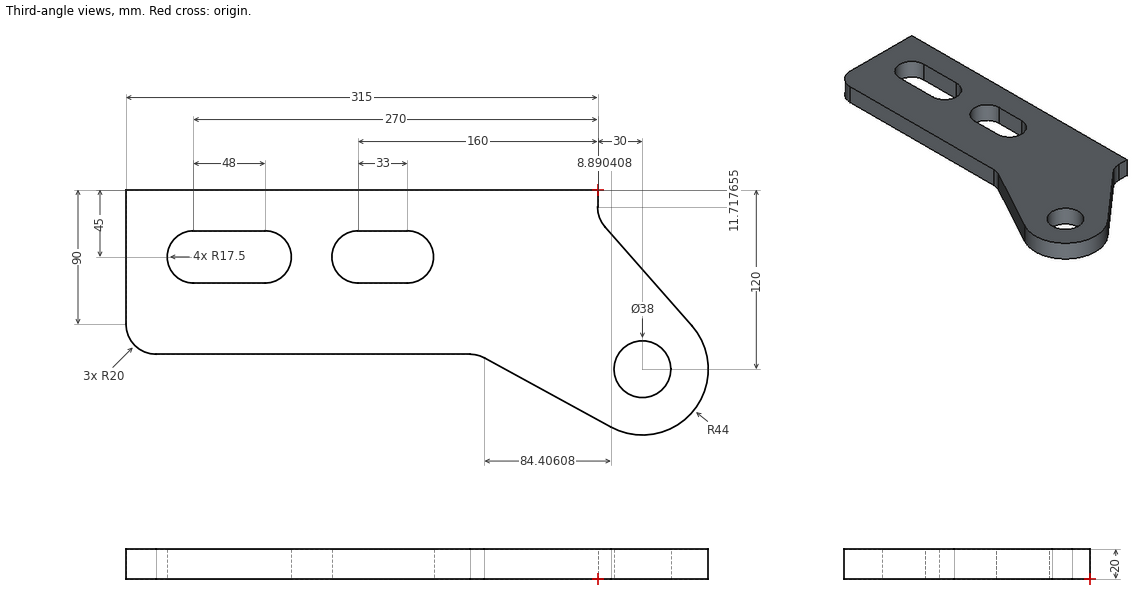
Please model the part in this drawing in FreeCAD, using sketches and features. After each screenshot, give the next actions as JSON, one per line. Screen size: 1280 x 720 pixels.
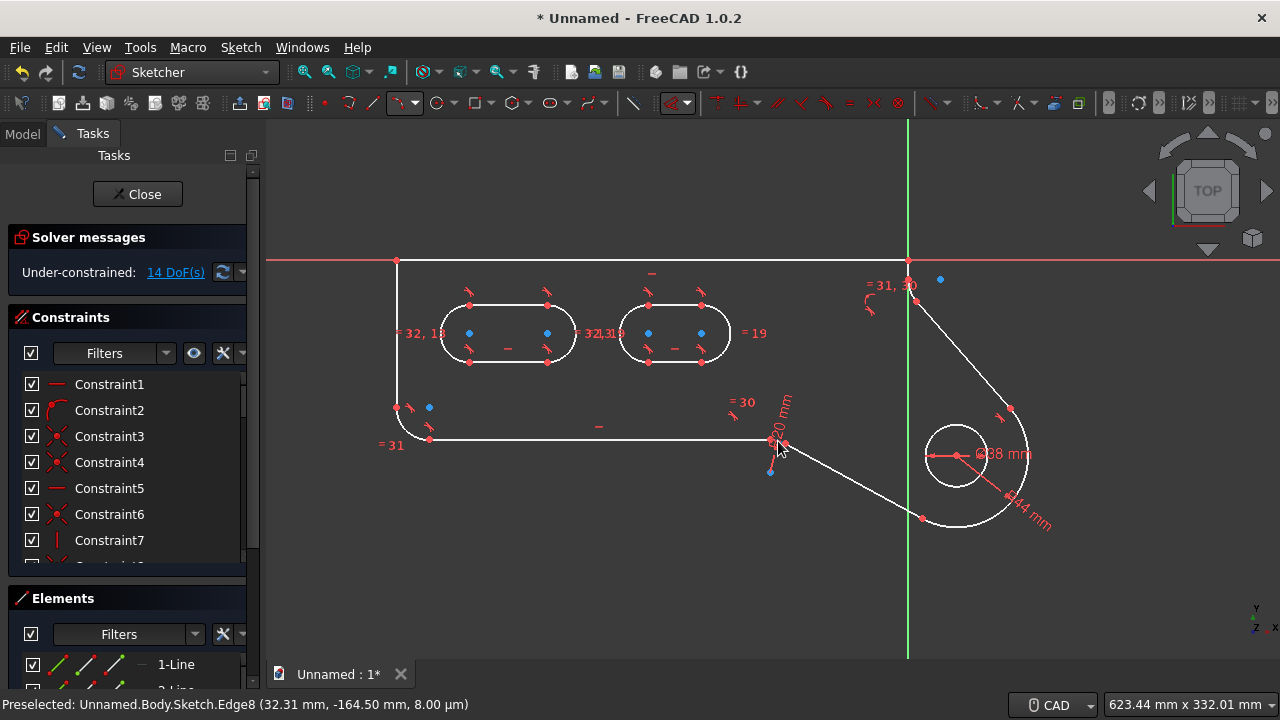
{"action": "scroll", "coordinate": [446, 317], "scroll_direction": "up", "scroll_amount": 2}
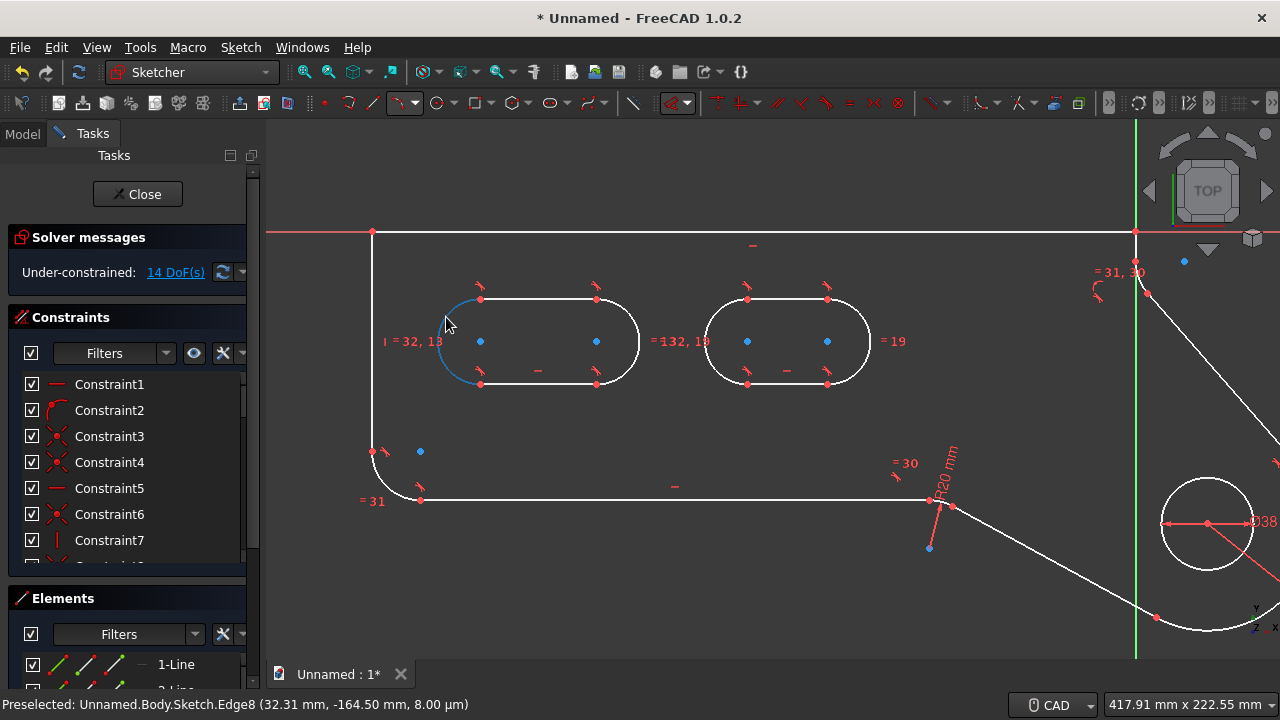
{"action": "left_click", "coordinate": [446, 317]}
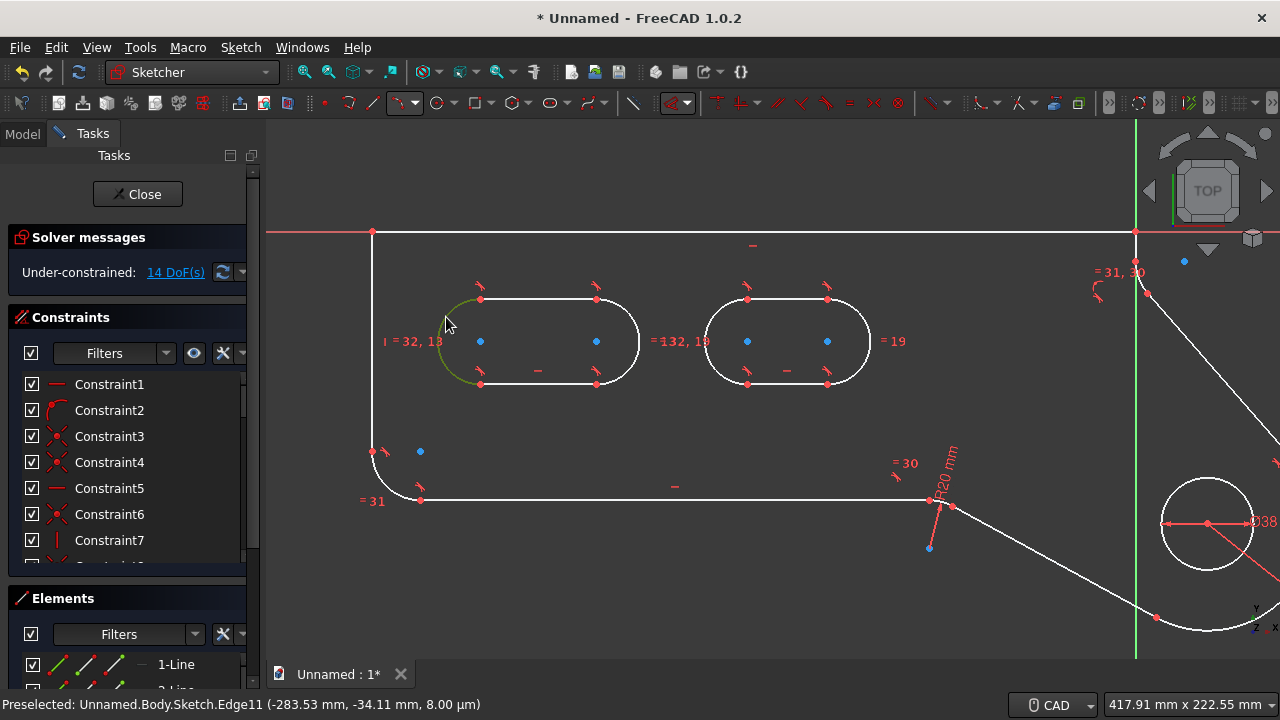
{"action": "key", "text": "k r"}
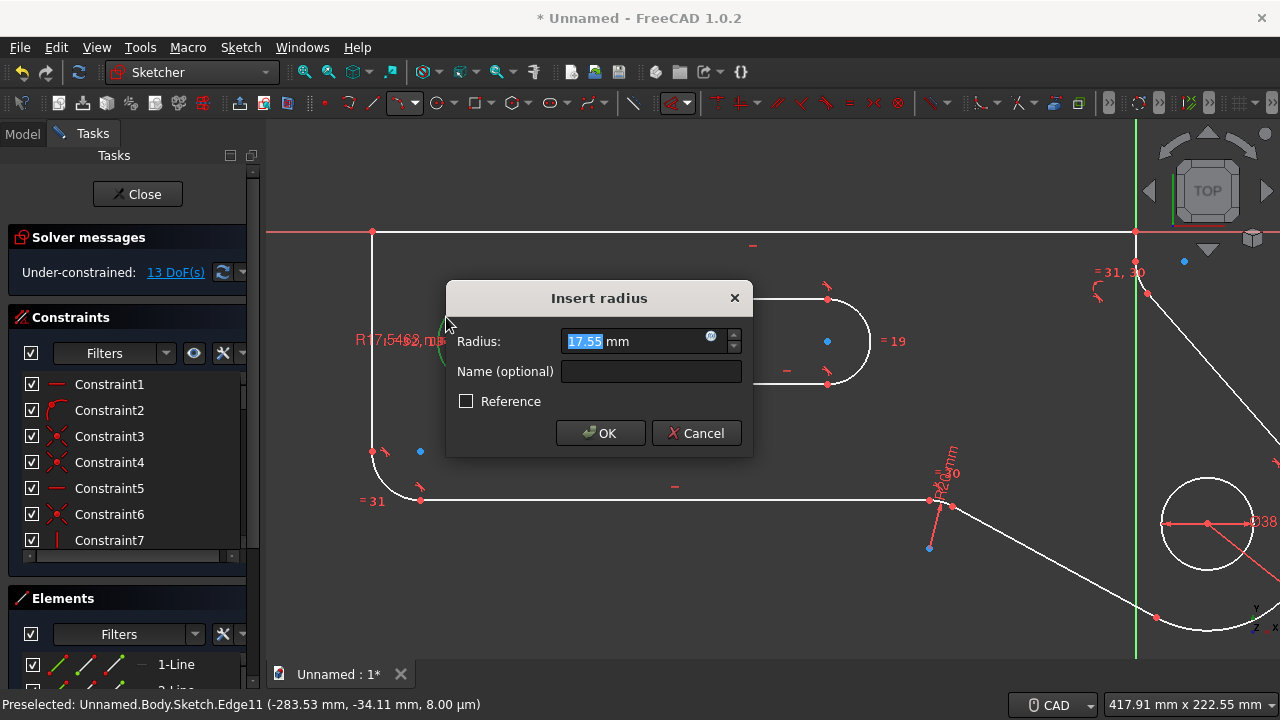
{"action": "type", "text": "17.5"}
{"action": "key", "text": "Return"}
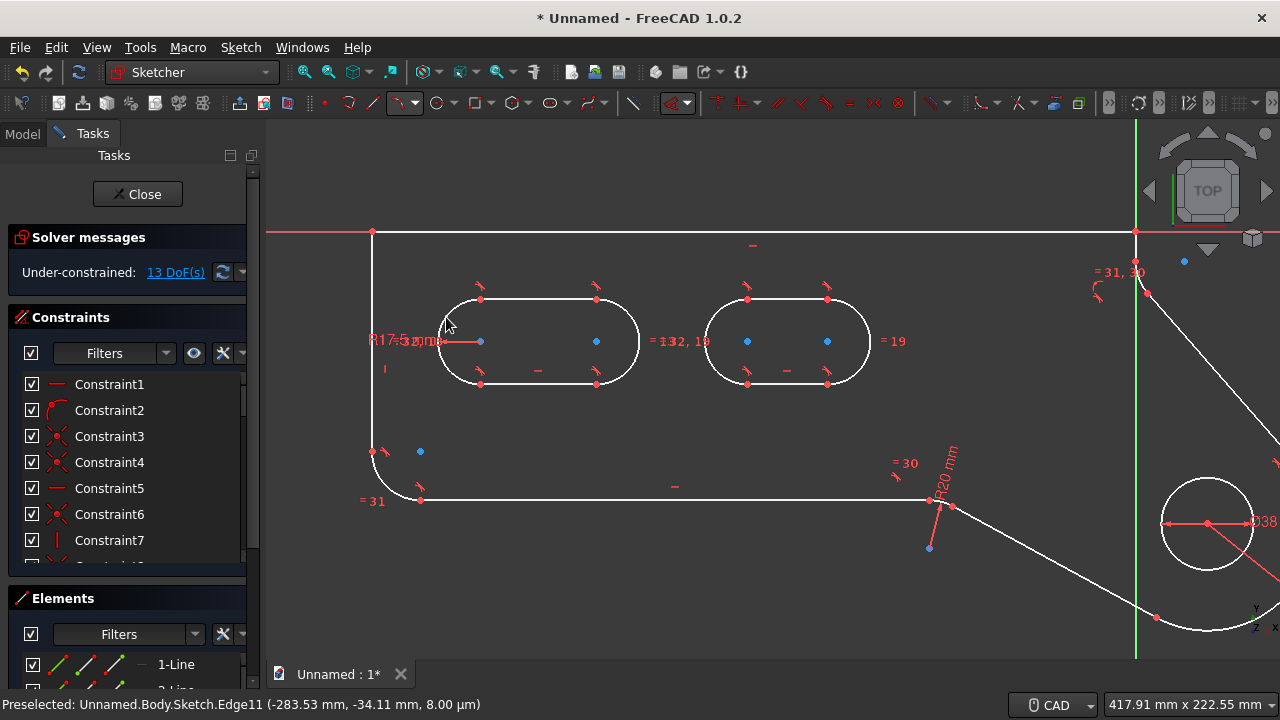
{"action": "left_click", "coordinate": [372, 298]}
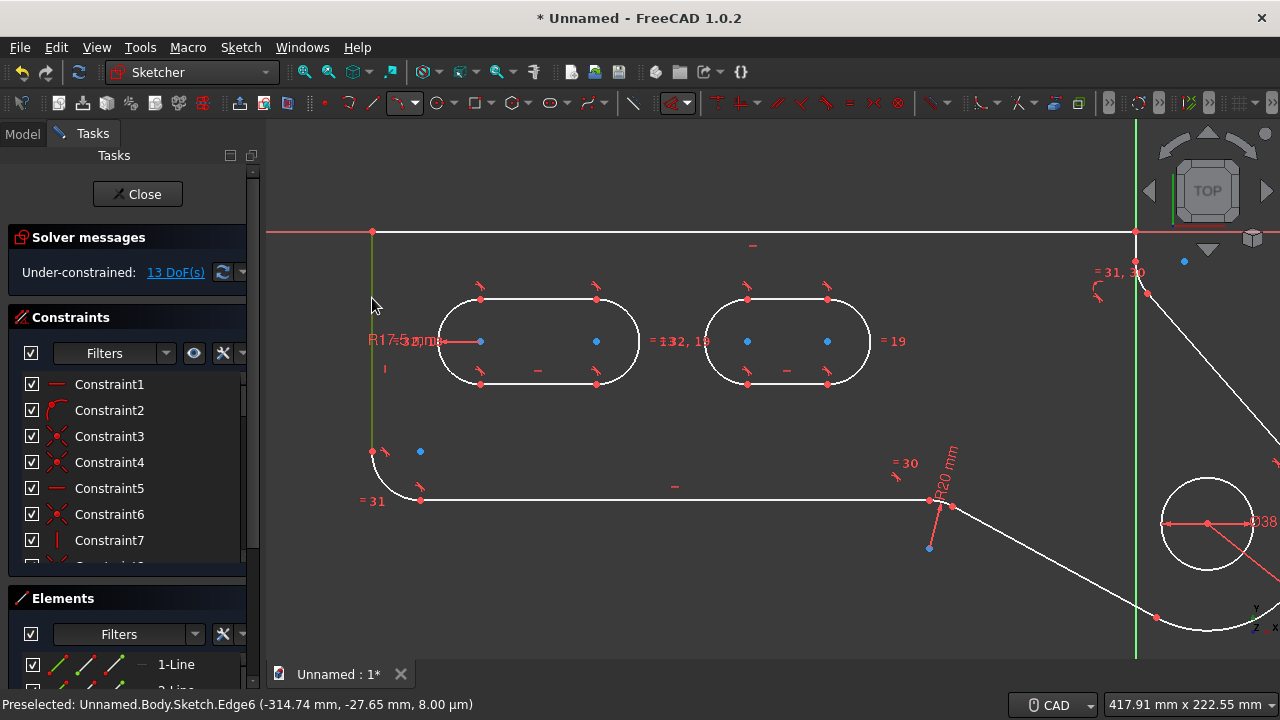
{"action": "key", "text": "i"}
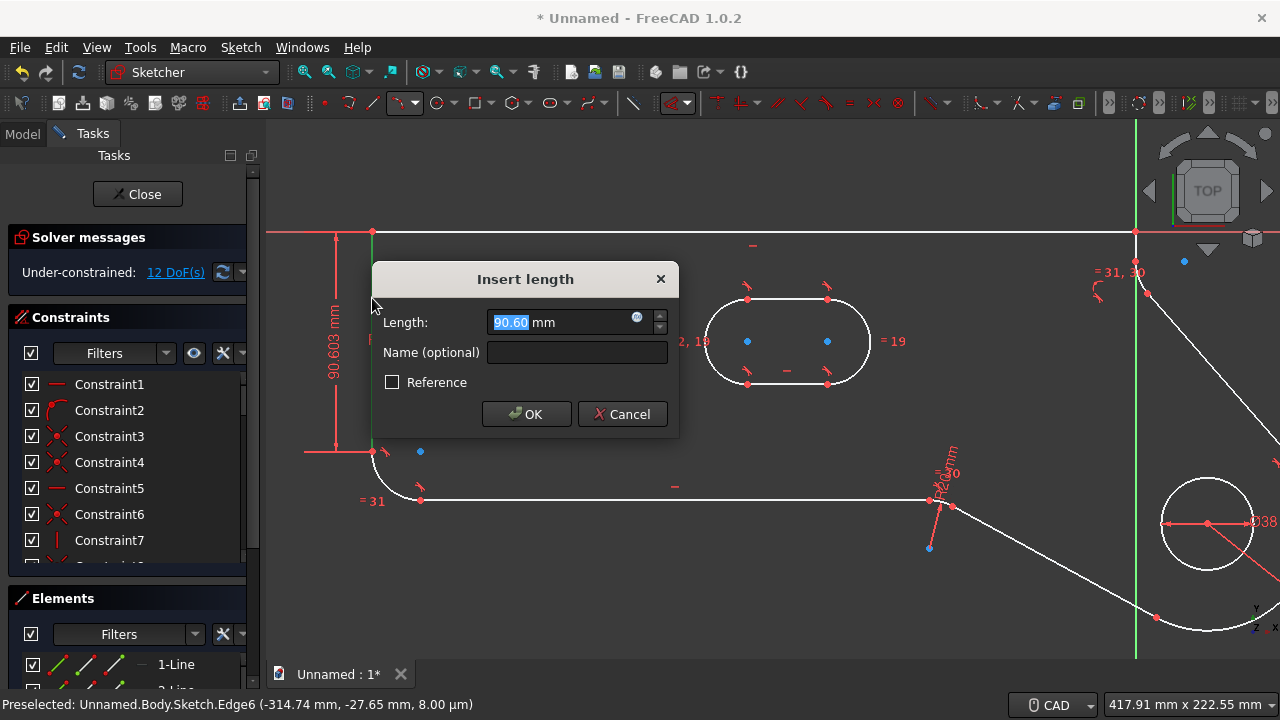
{"action": "type", "text": "90"}
{"action": "key", "text": "Return"}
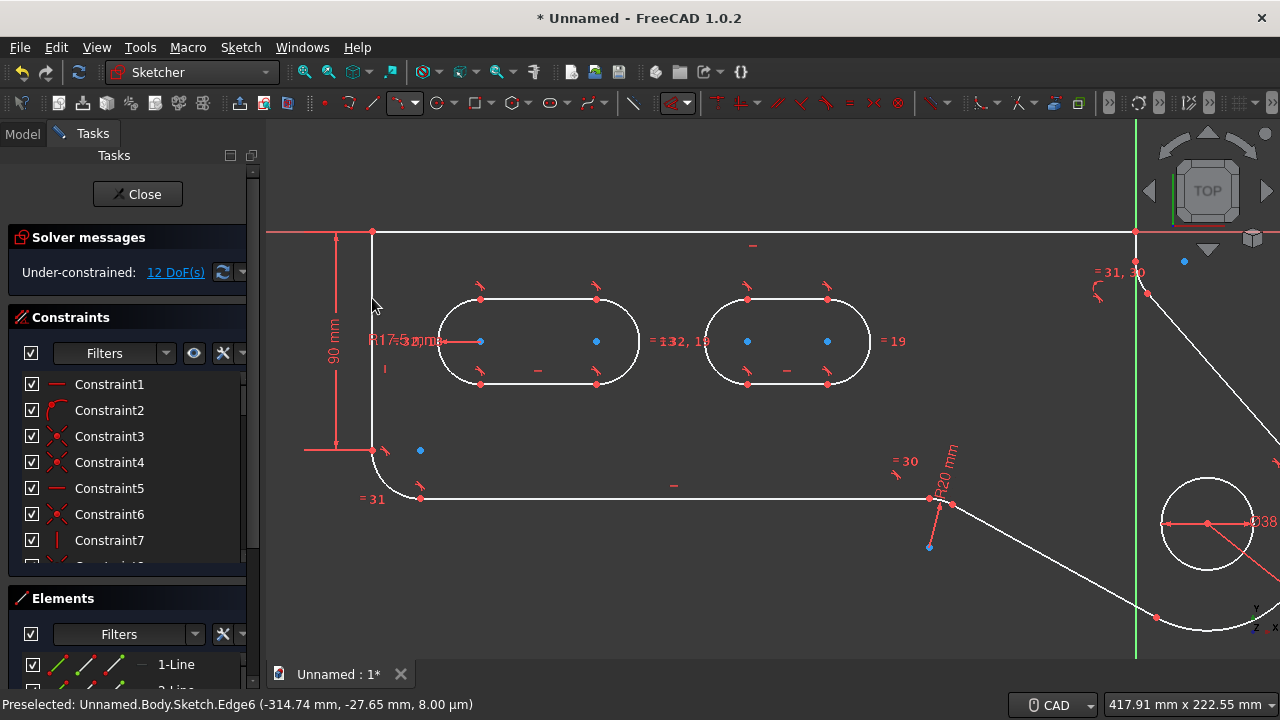
{"action": "left_click", "coordinate": [516, 299]}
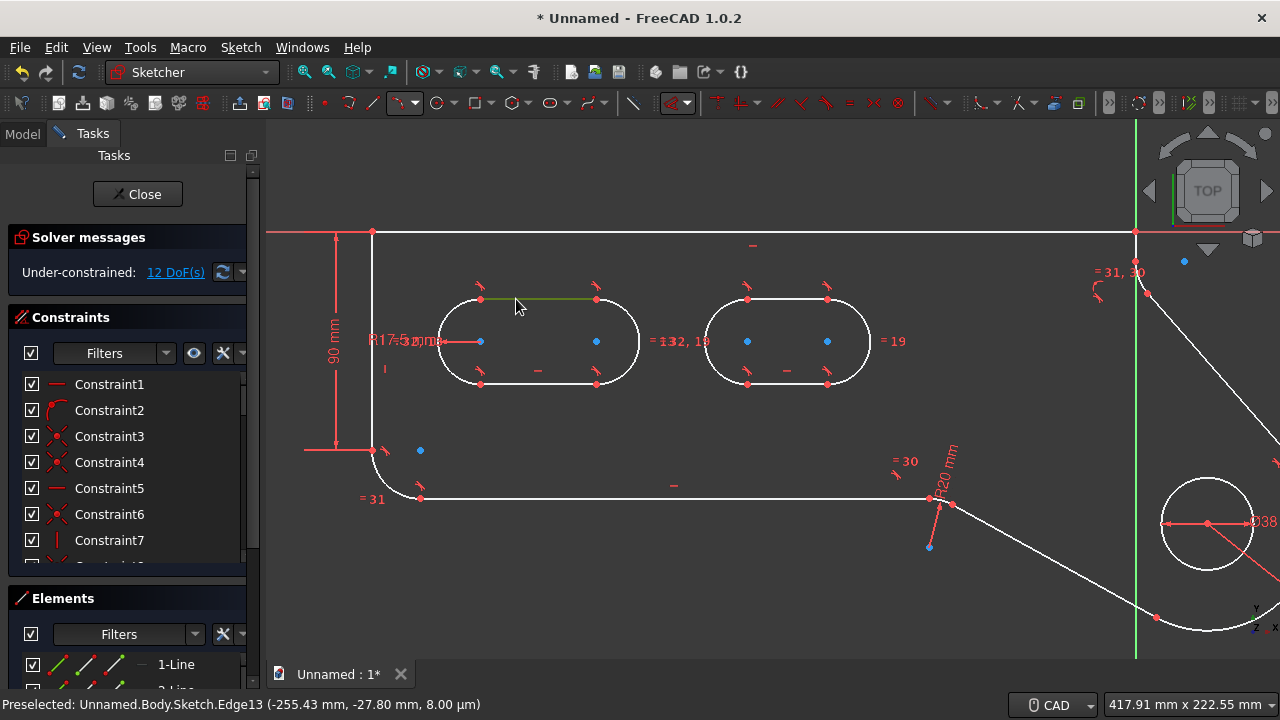
{"action": "key", "text": "l"}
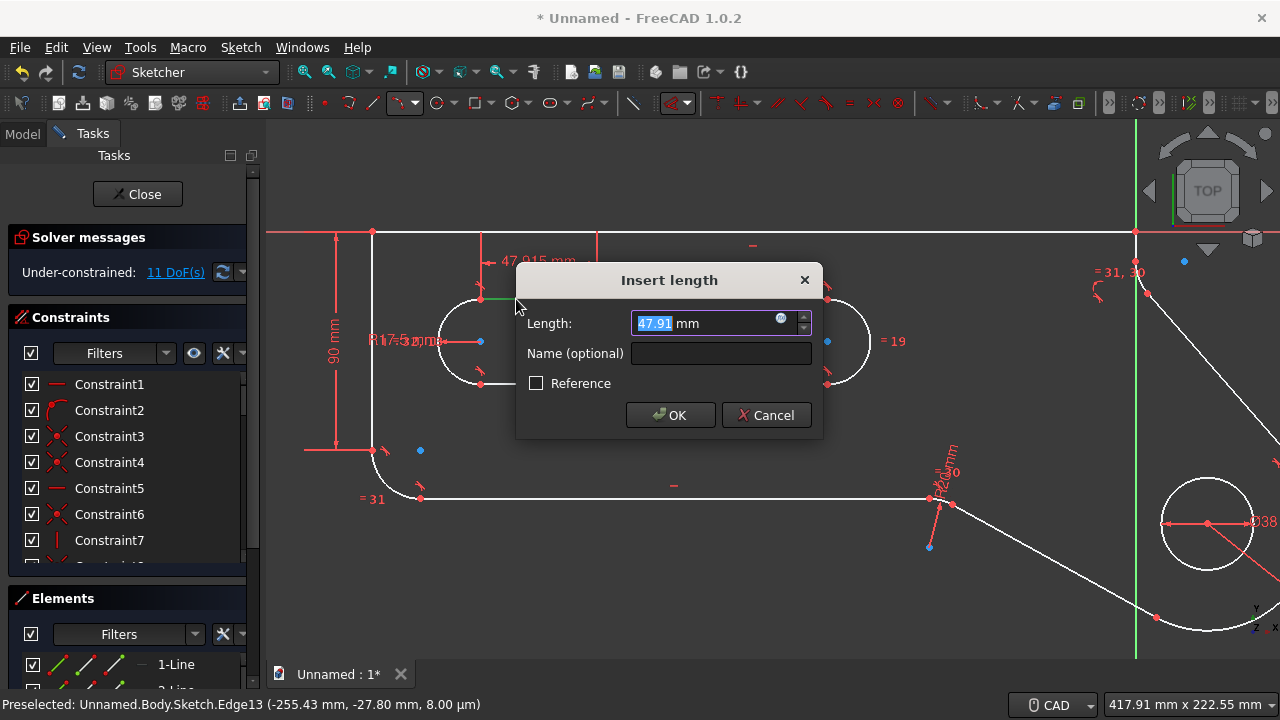
{"action": "type", "text": "48"}
{"action": "key", "text": "Return"}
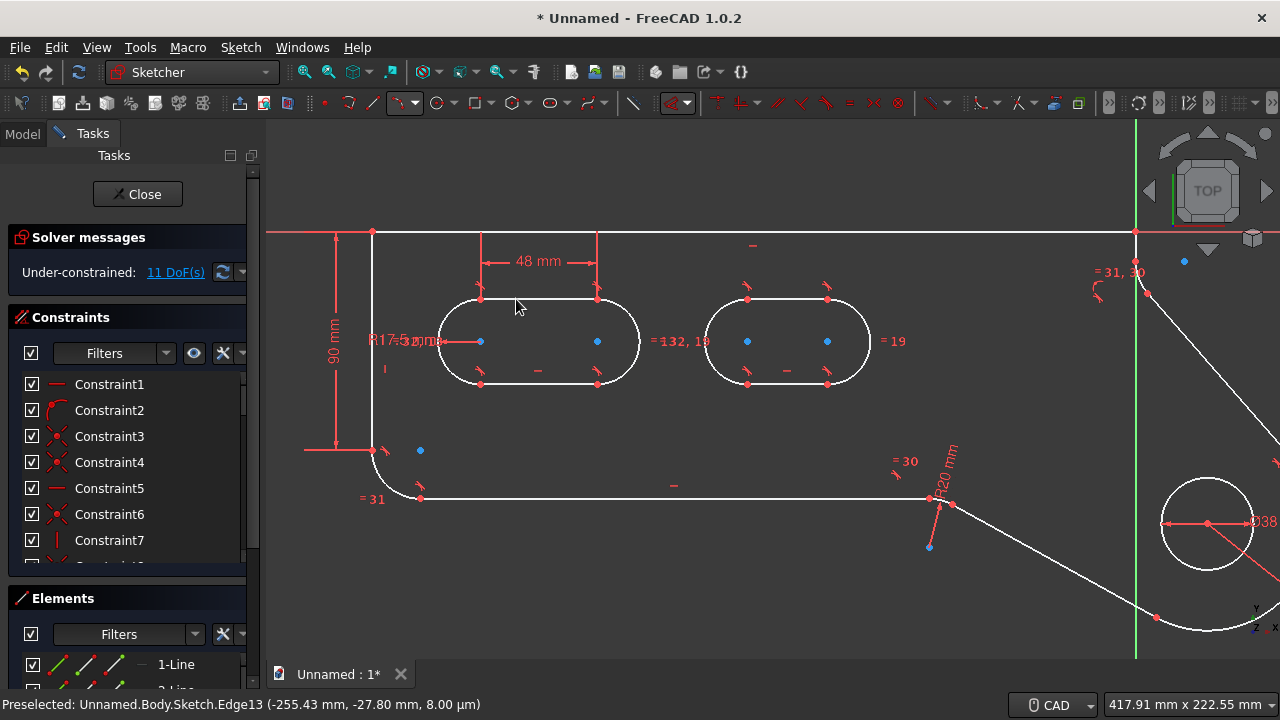
{"action": "left_click", "coordinate": [772, 299]}